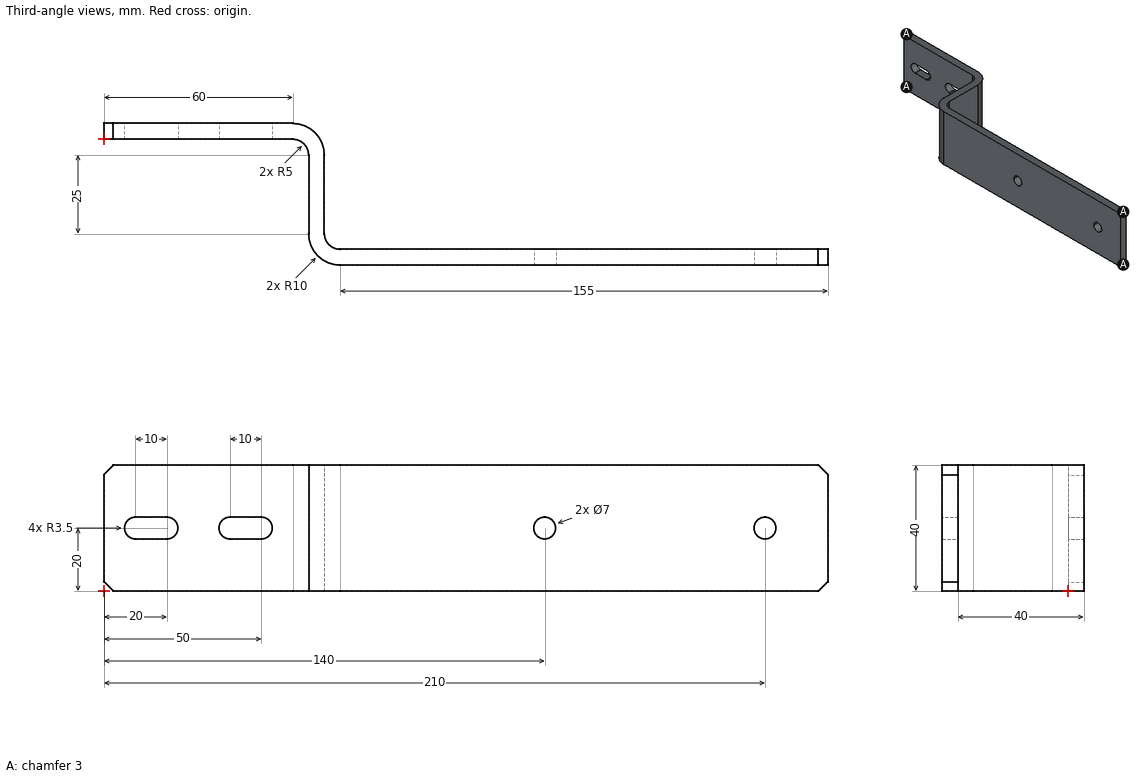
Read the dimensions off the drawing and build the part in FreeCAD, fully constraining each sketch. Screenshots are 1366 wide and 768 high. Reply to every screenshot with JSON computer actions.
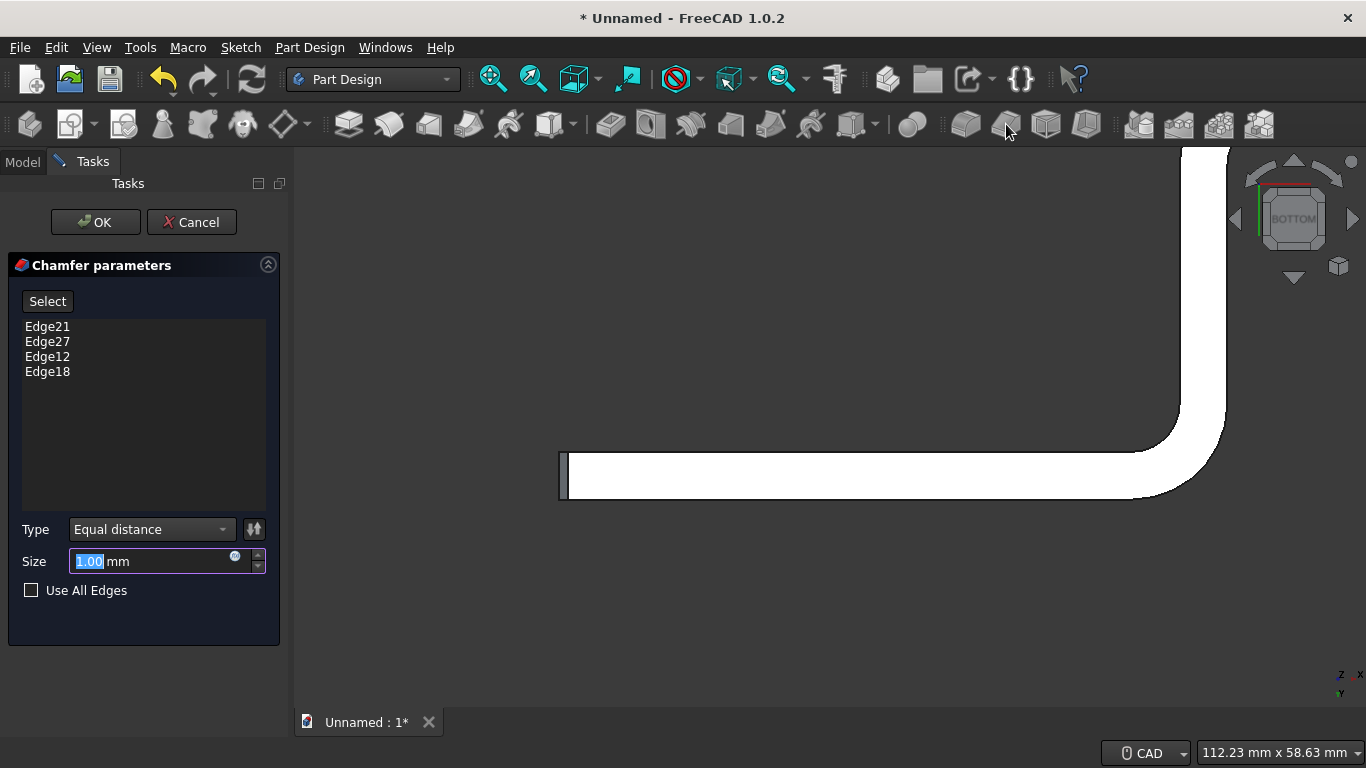
{"action": "type", "text": "3"}
{"action": "key", "text": "Tab"}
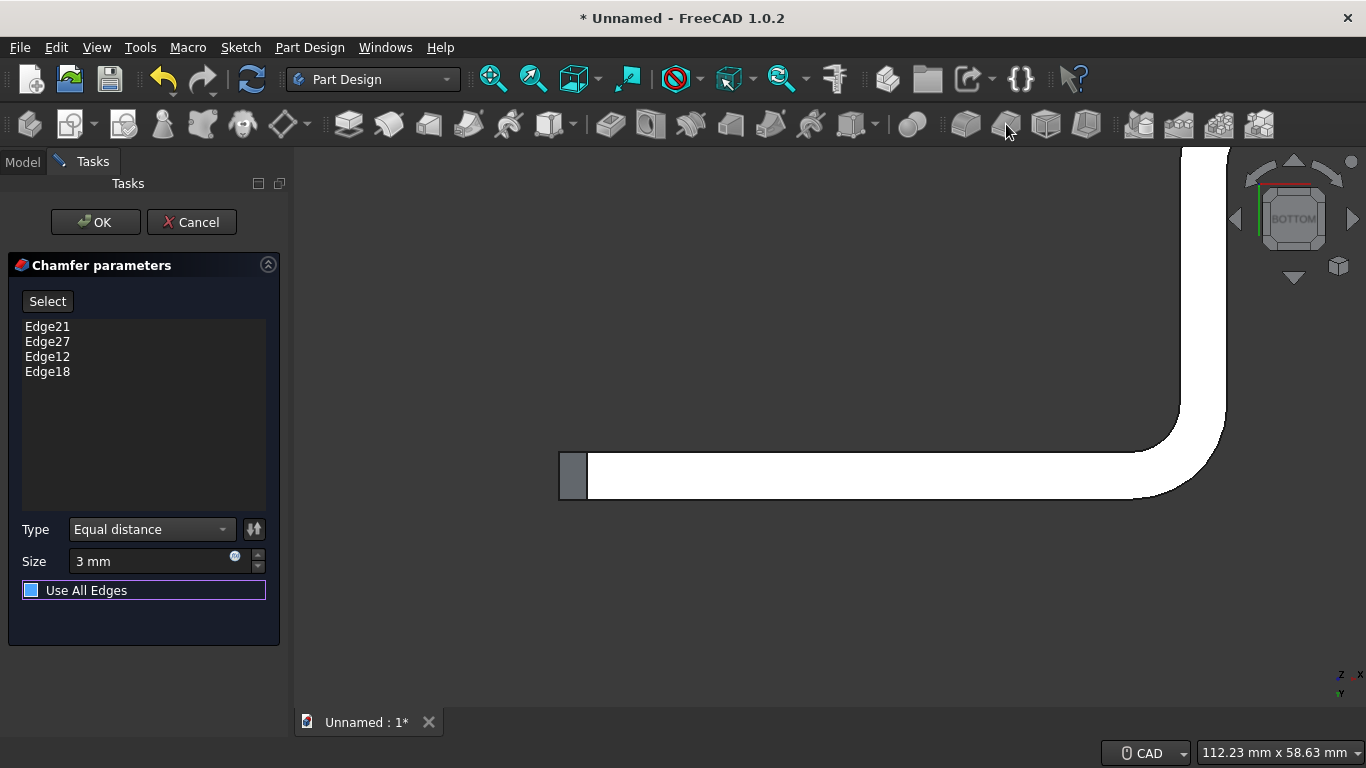
{"action": "left_click", "coordinate": [96, 222]}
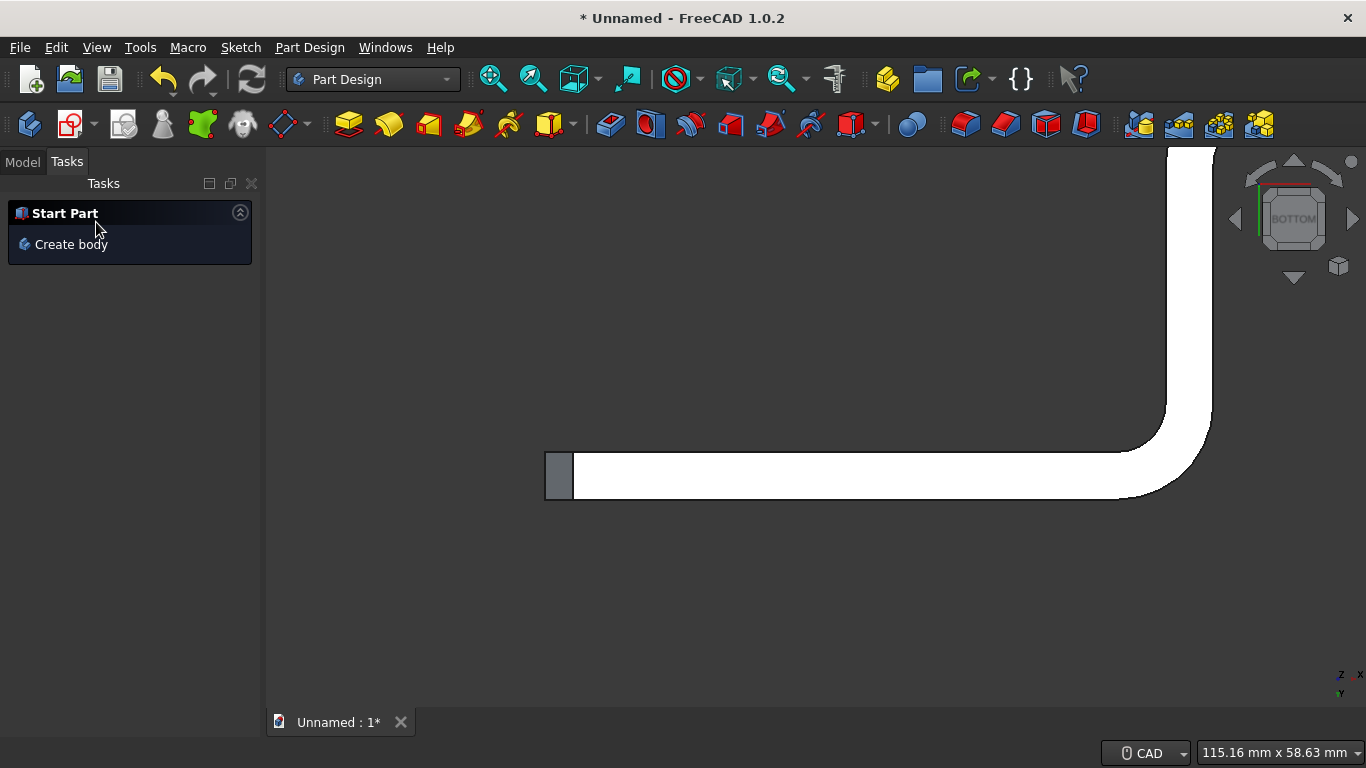
{"action": "key", "text": "0"}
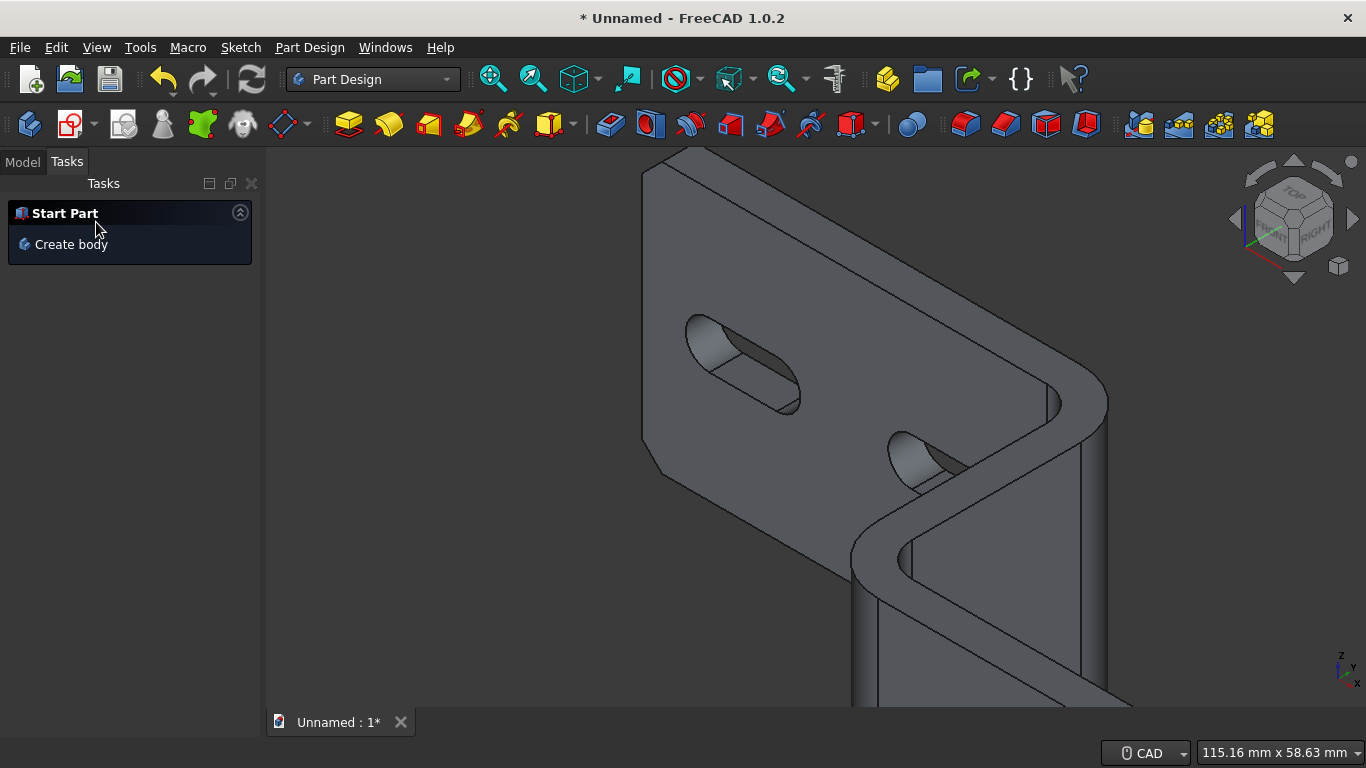
{"action": "left_click", "coordinate": [494, 80]}